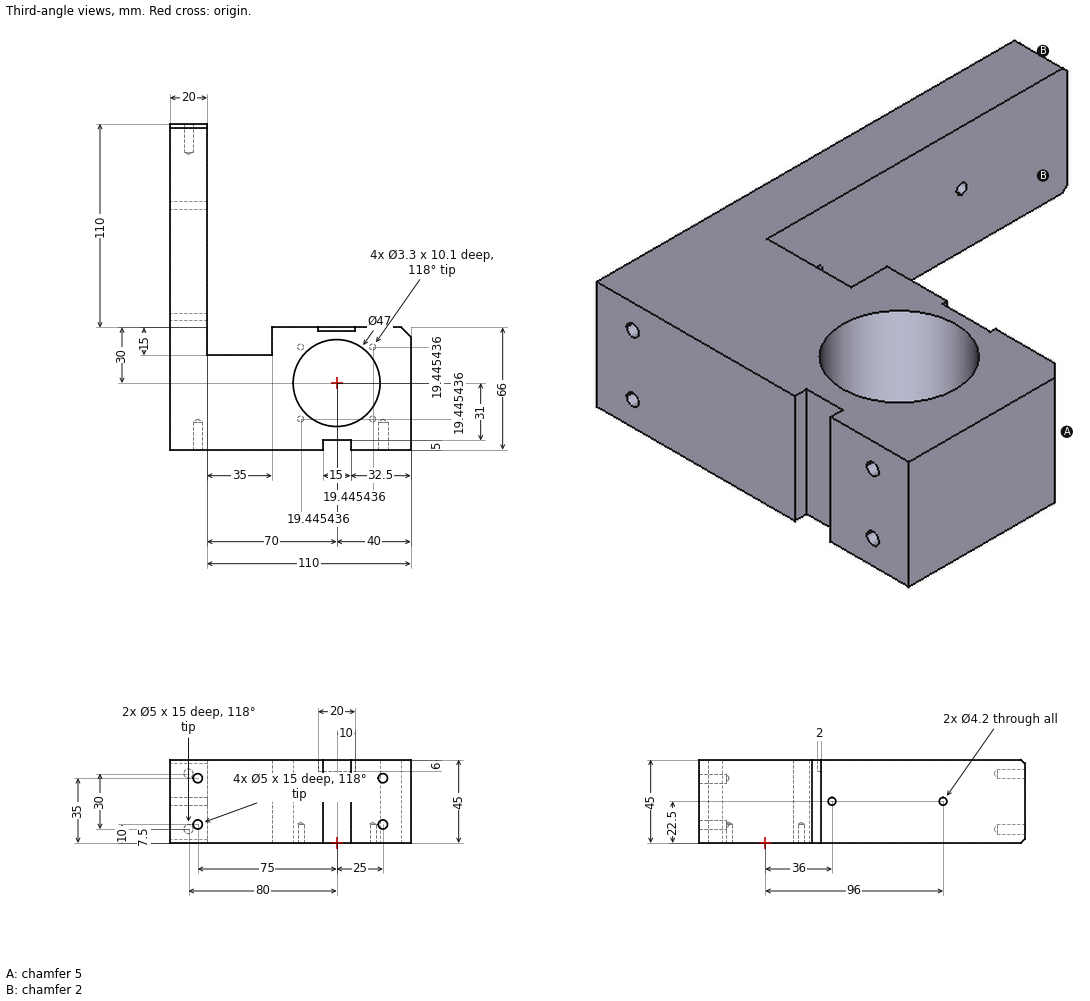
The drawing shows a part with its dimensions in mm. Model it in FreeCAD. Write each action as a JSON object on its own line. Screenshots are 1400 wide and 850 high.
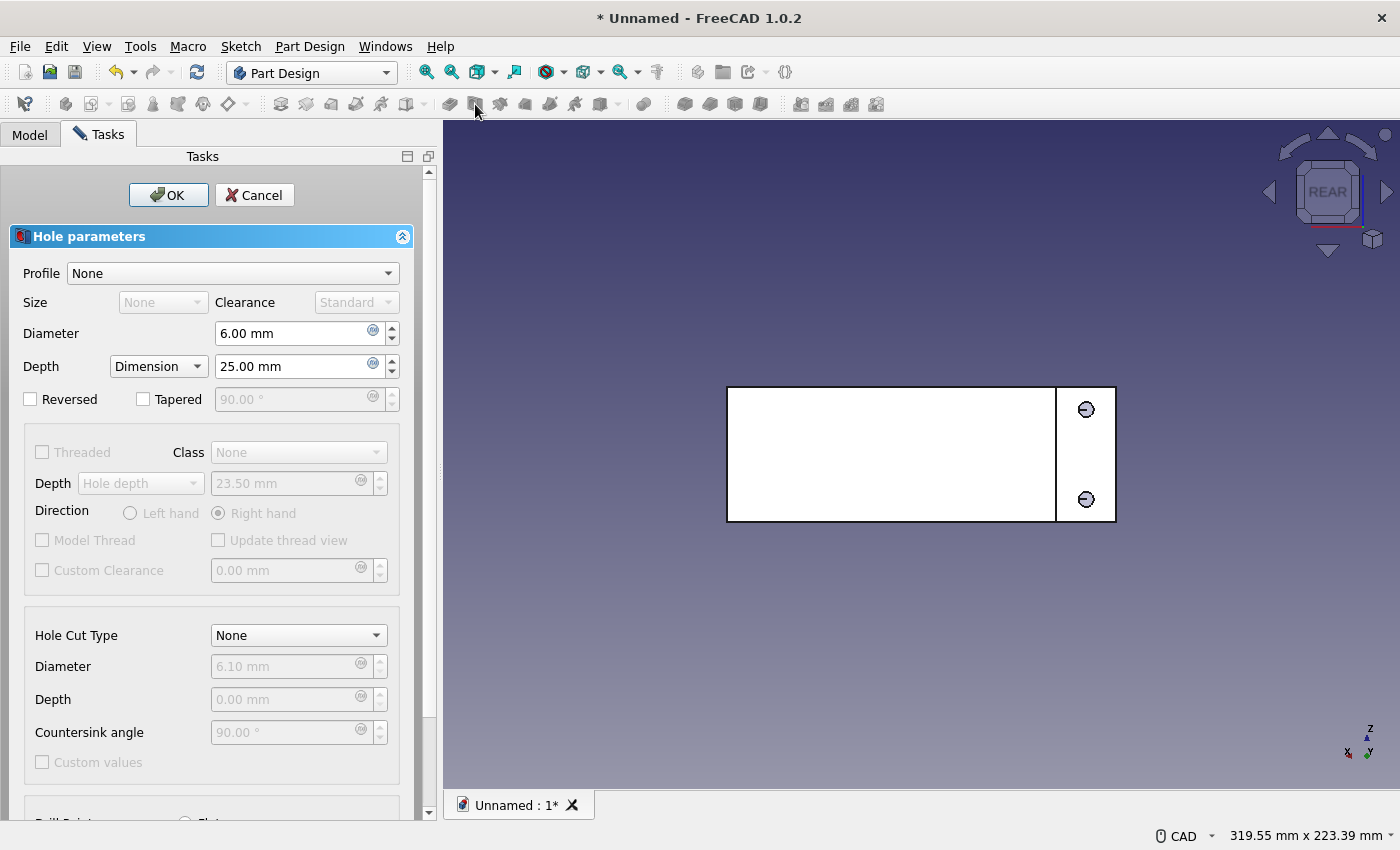
{"action": "triple_click", "coordinate": [300, 334]}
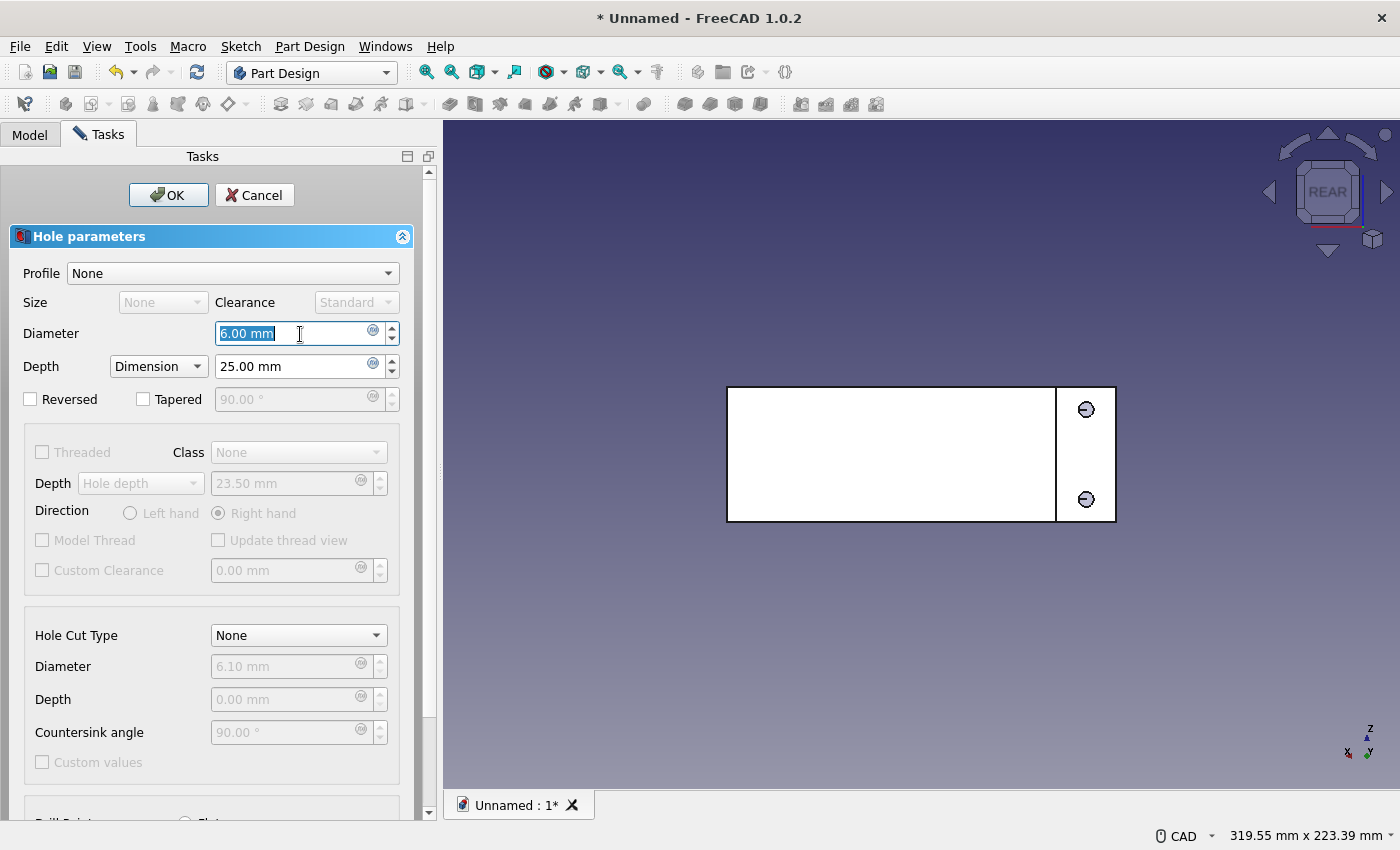
{"action": "type", "text": "3.3"}
{"action": "key", "text": "Tab"}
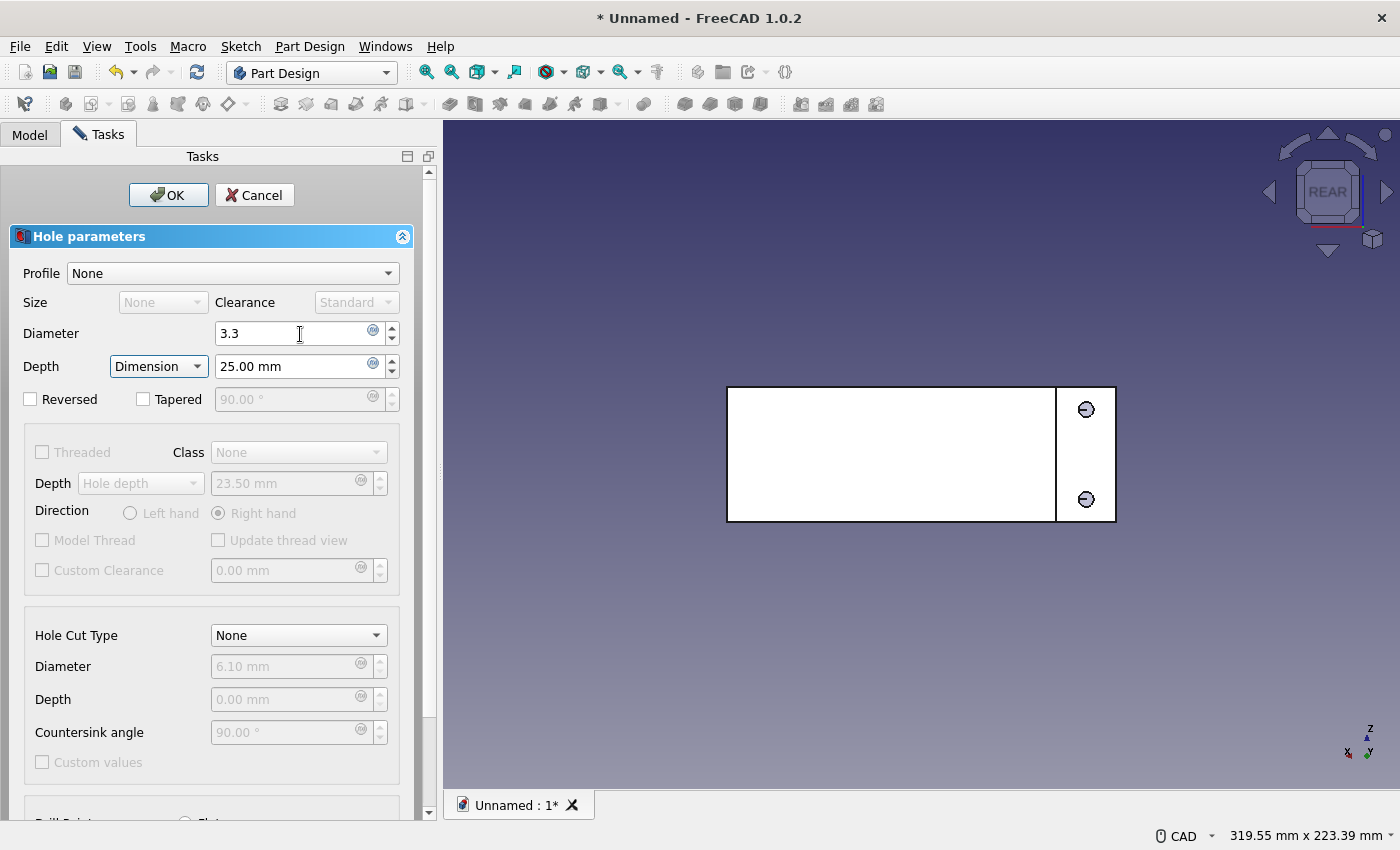
{"action": "triple_click", "coordinate": [300, 366]}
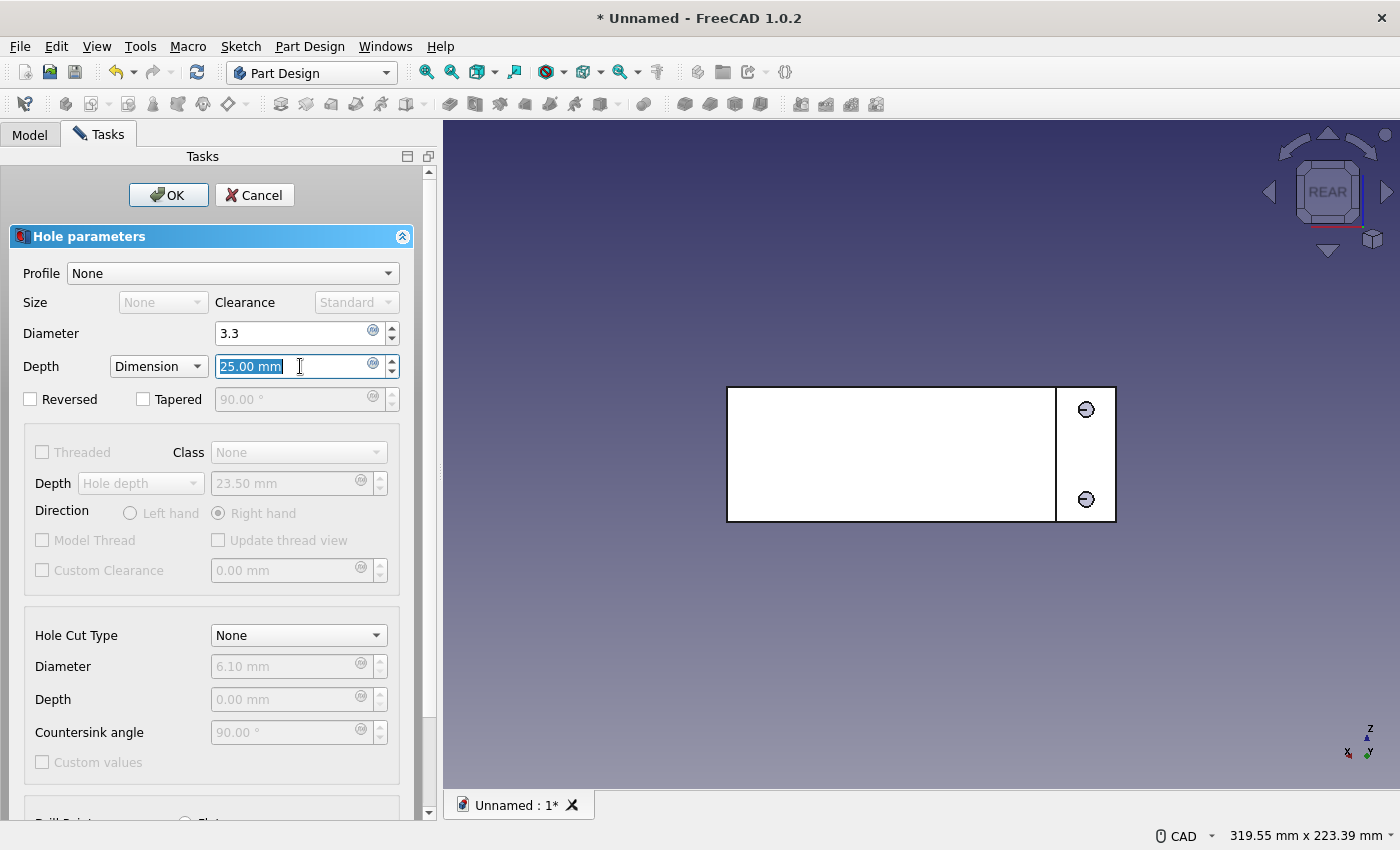
{"action": "type", "text": "10.1"}
{"action": "key", "text": "Tab"}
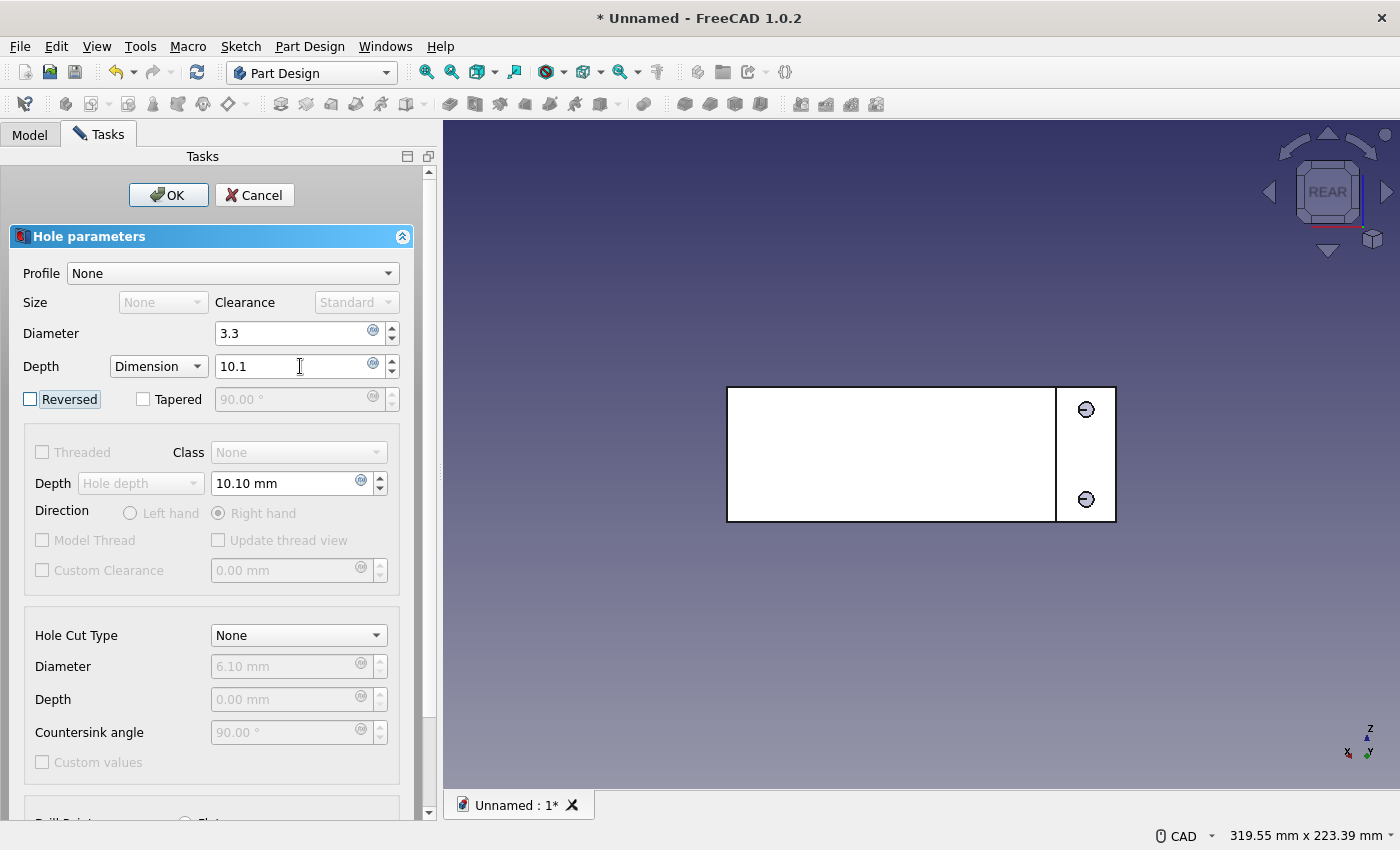
{"action": "left_click", "coordinate": [31, 399]}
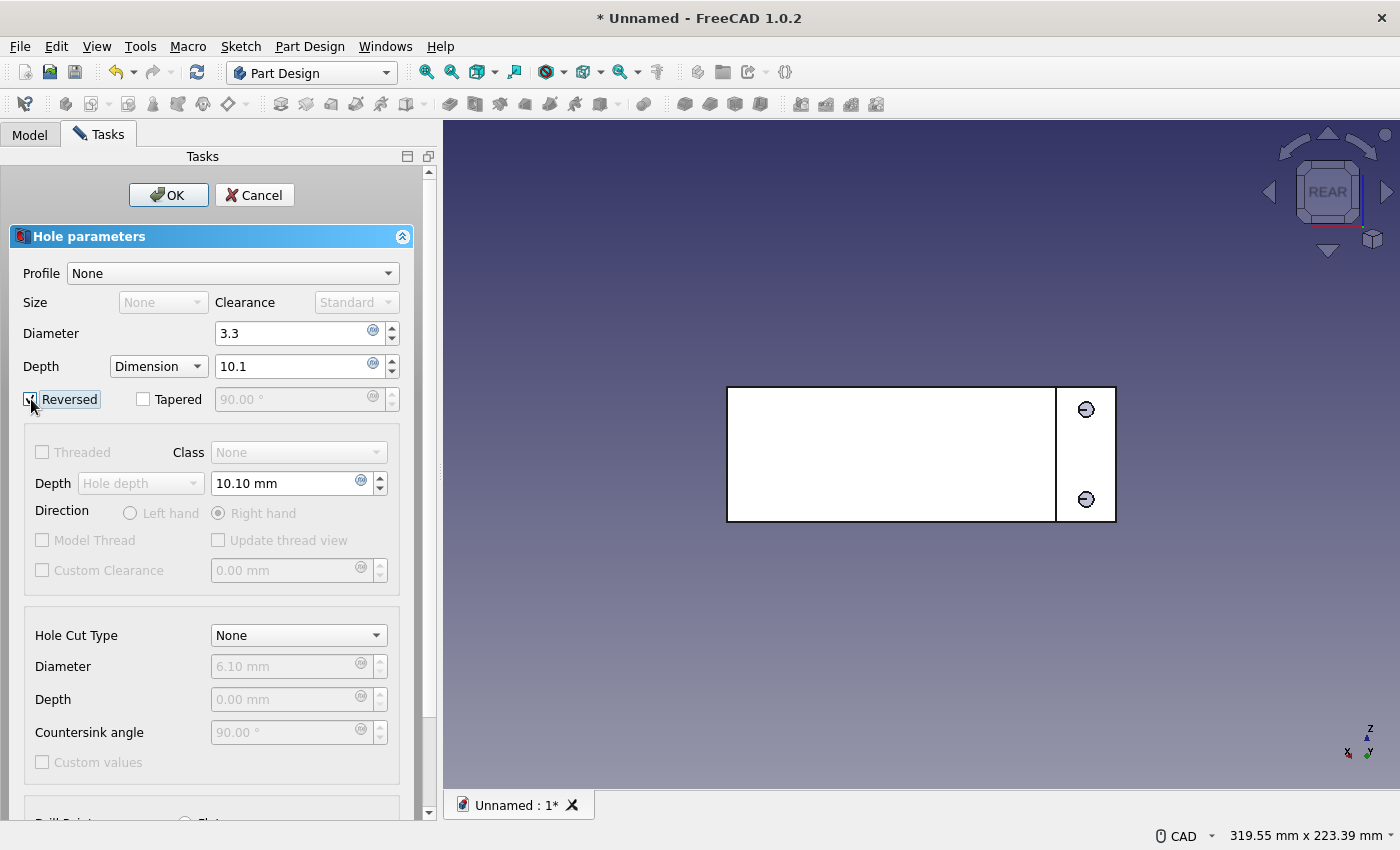
{"action": "left_click", "coordinate": [169, 195]}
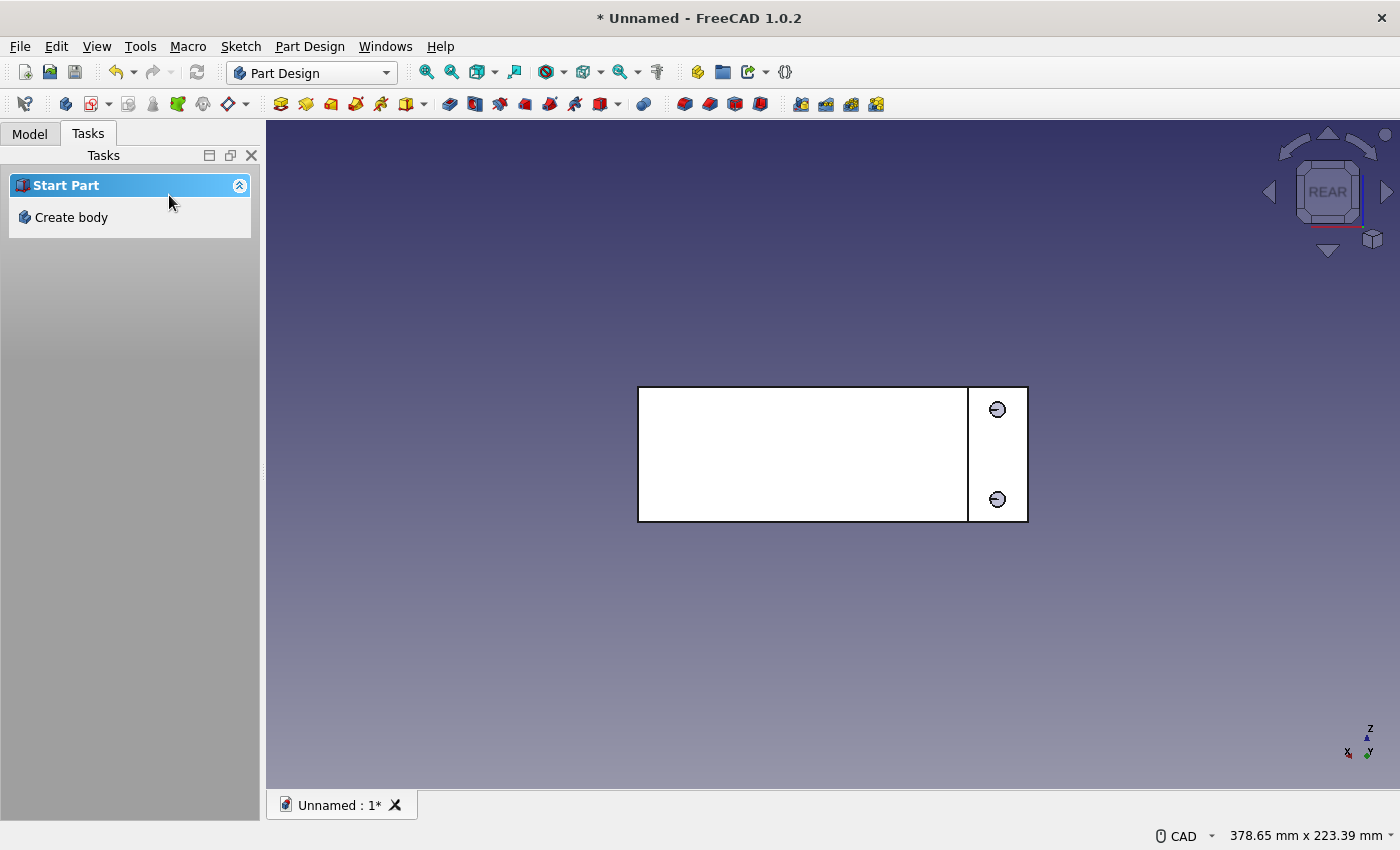
{"action": "left_click", "coordinate": [427, 72]}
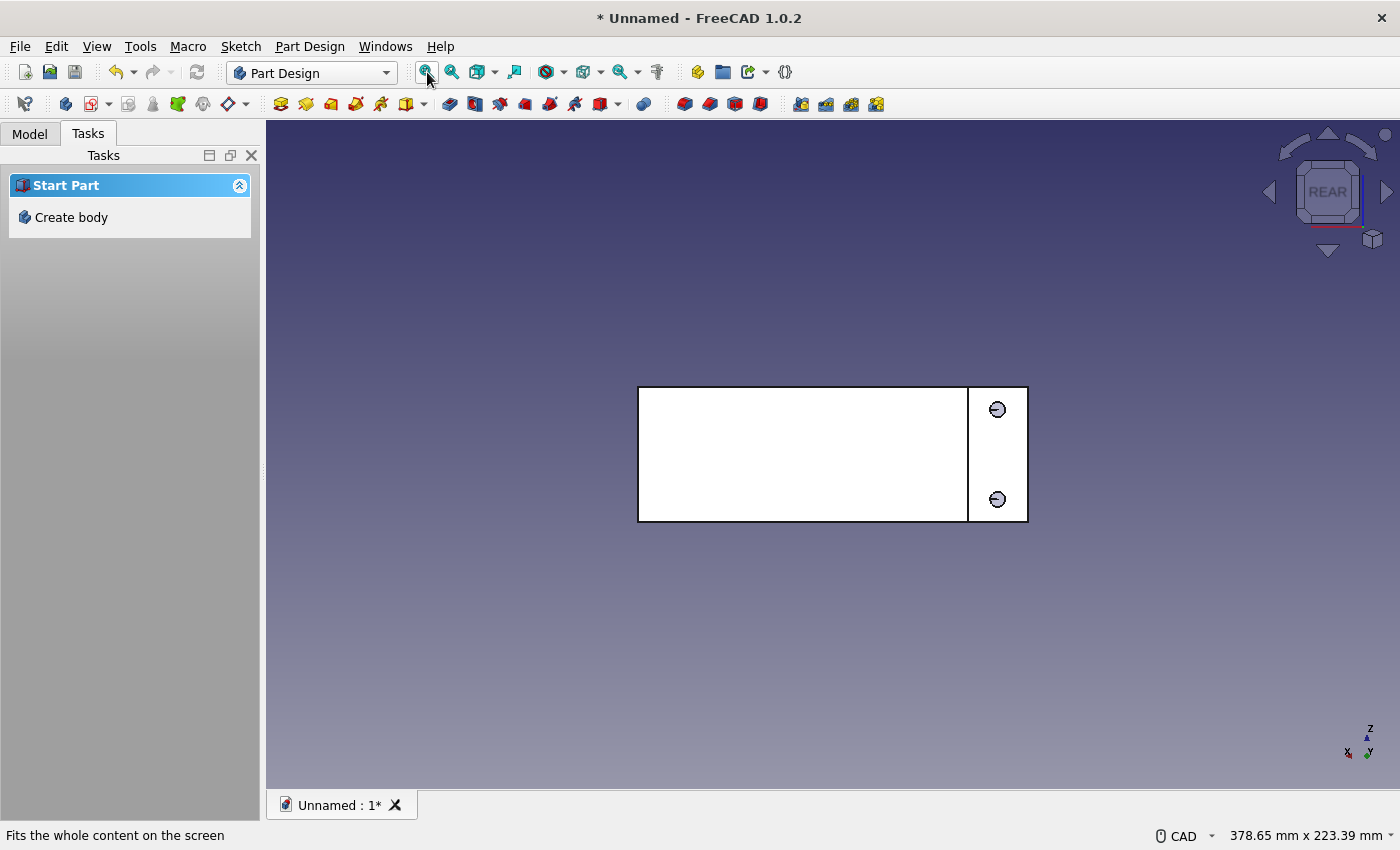
{"action": "key", "text": "0"}